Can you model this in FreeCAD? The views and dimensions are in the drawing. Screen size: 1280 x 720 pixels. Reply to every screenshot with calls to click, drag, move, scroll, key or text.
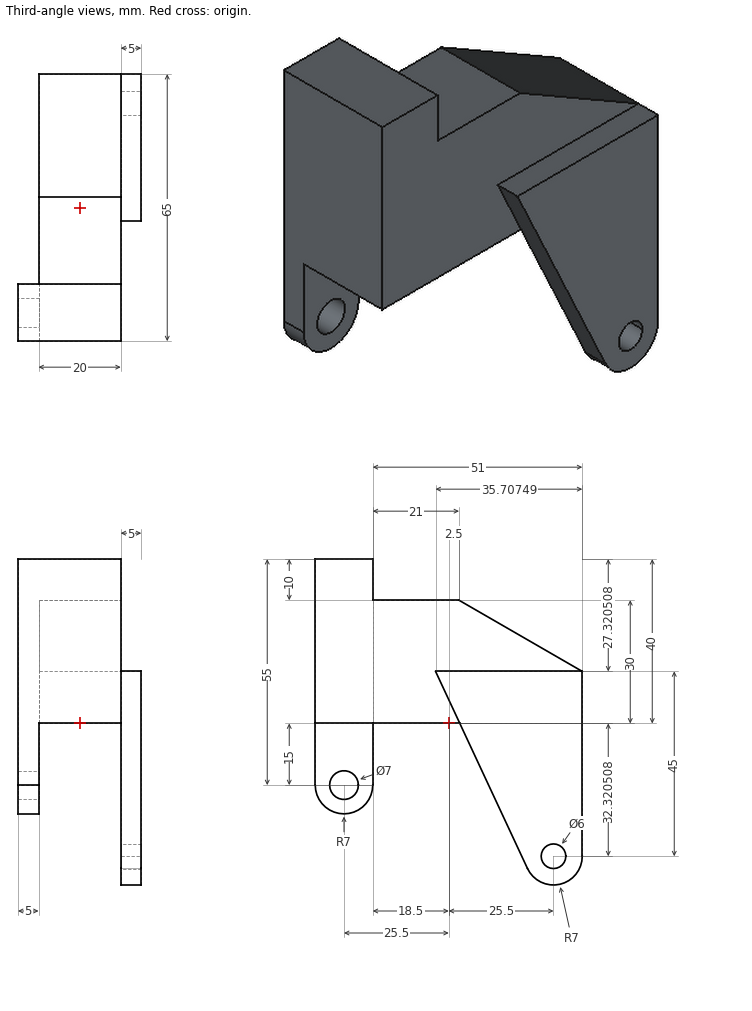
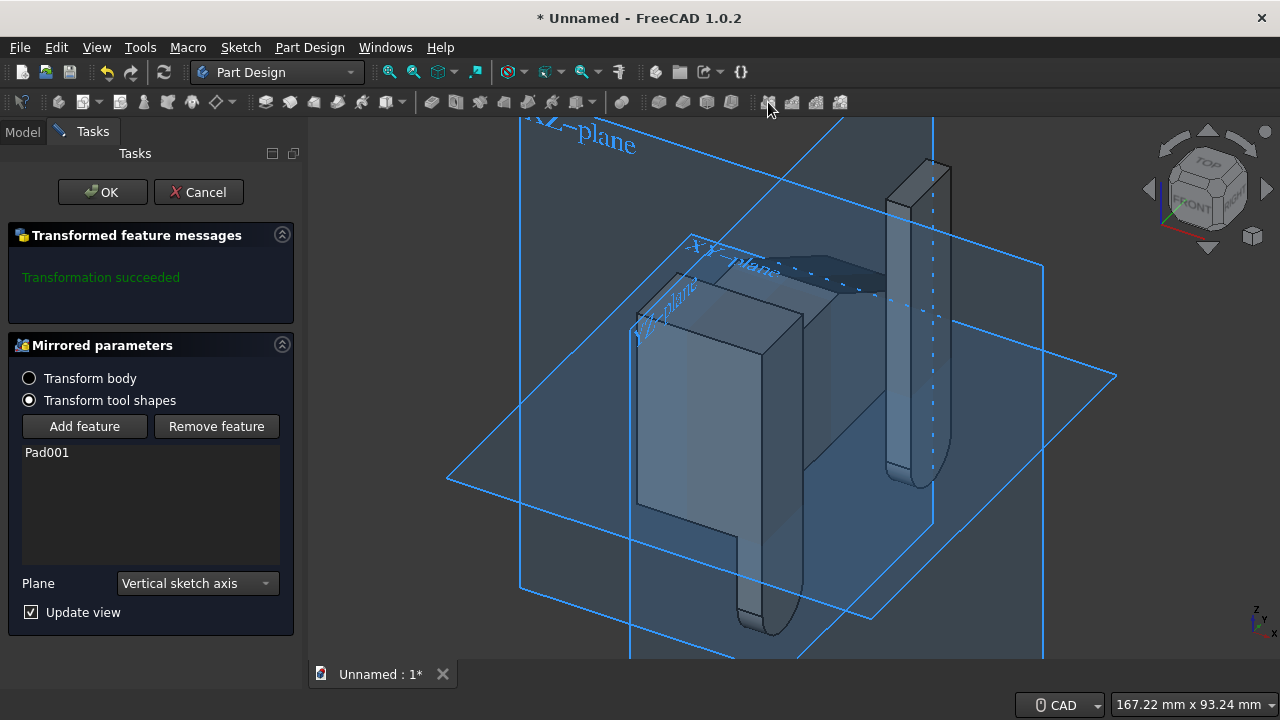
click(198, 584)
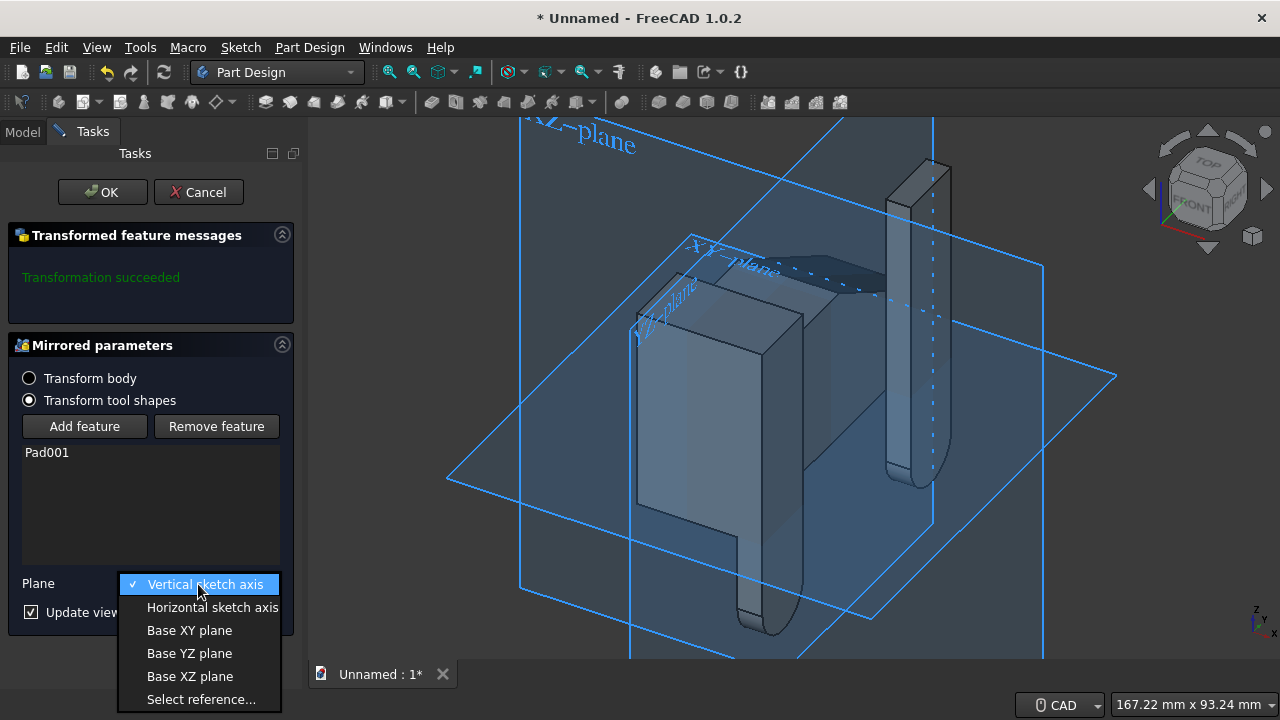
click(198, 654)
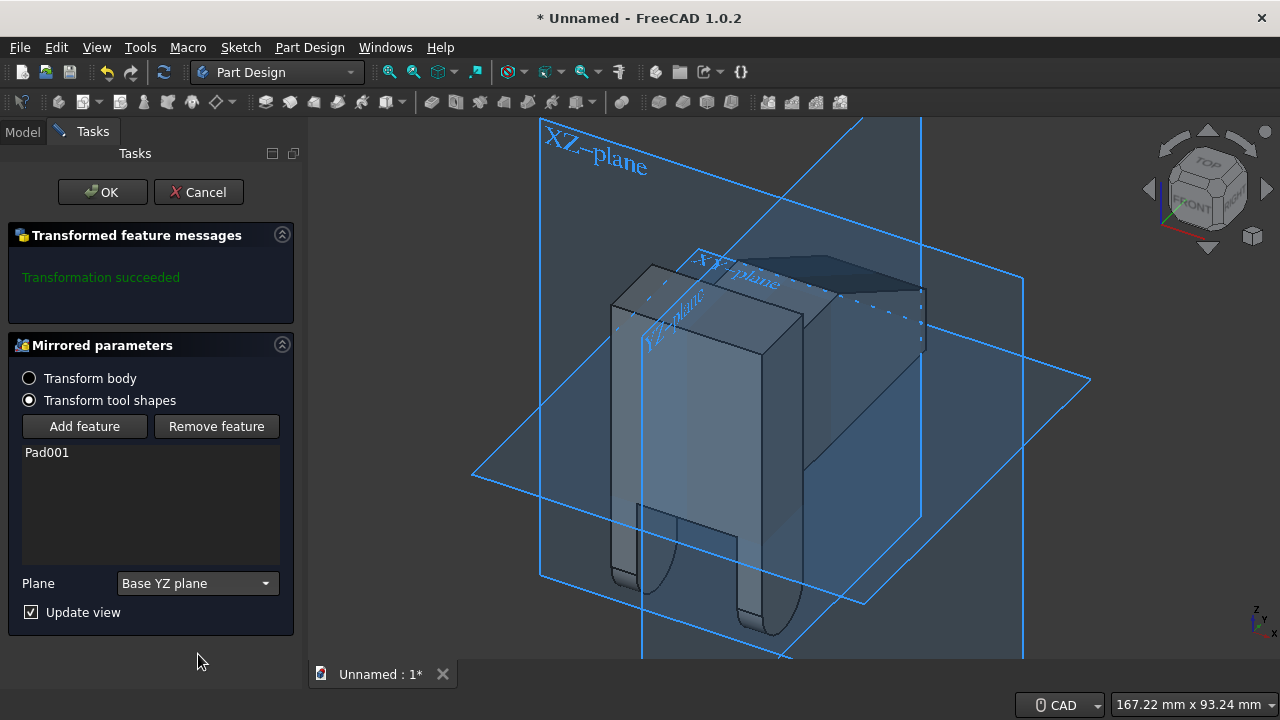
click(103, 192)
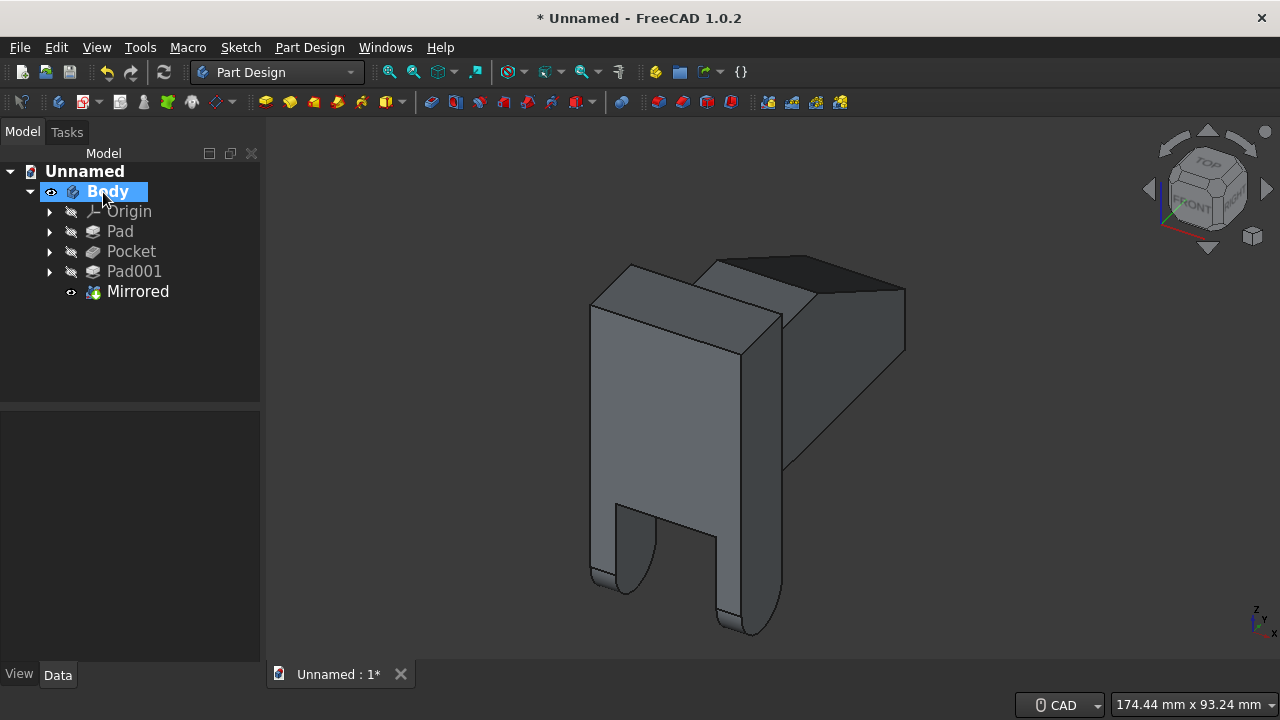
click(390, 72)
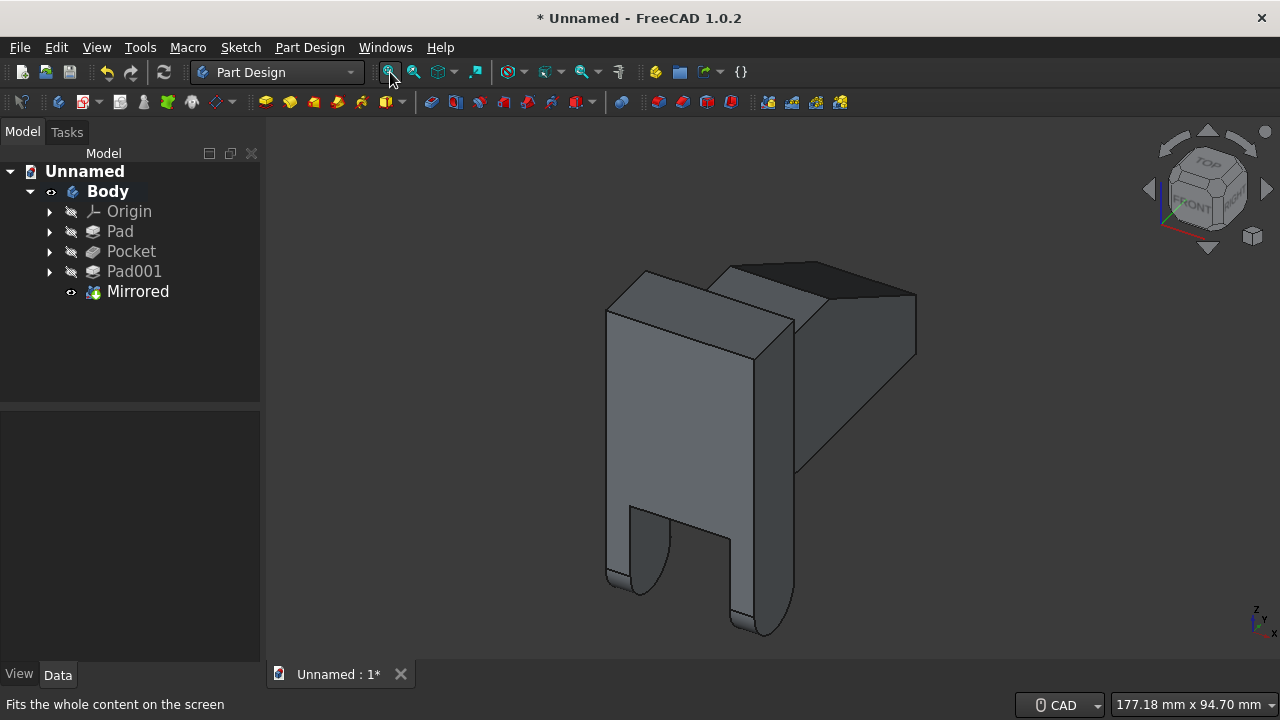
click(774, 401)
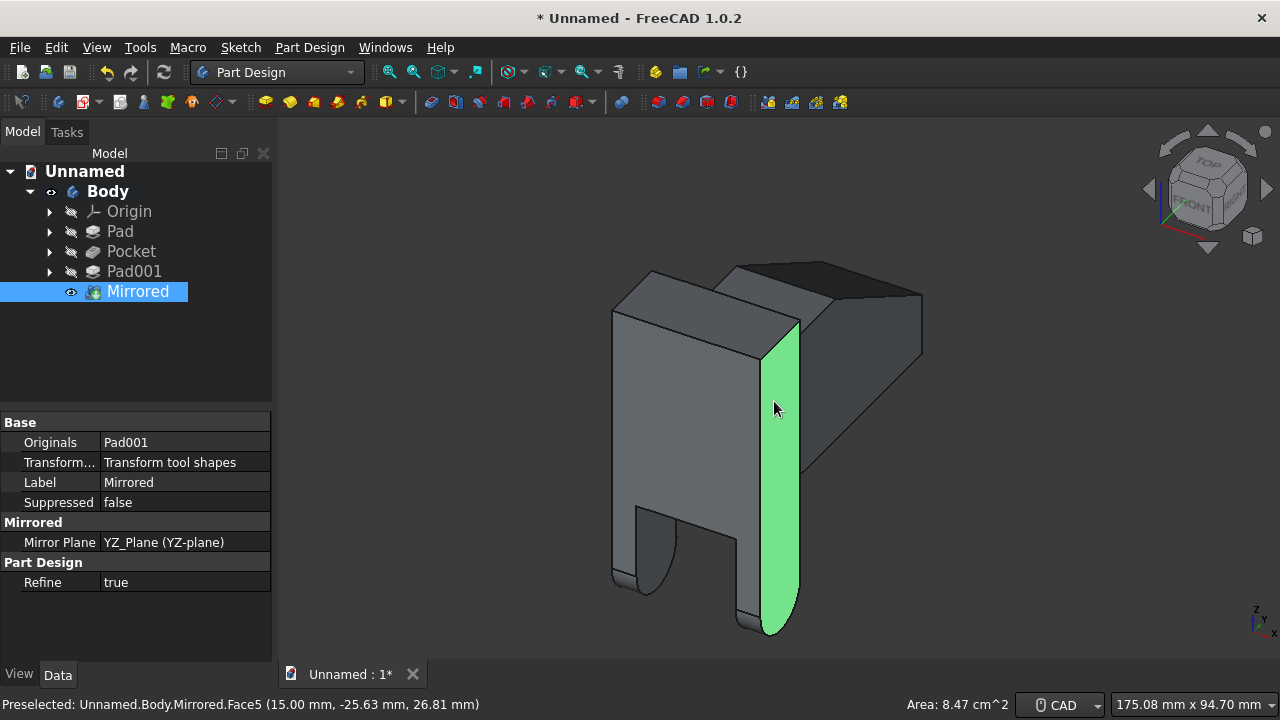
click(84, 102)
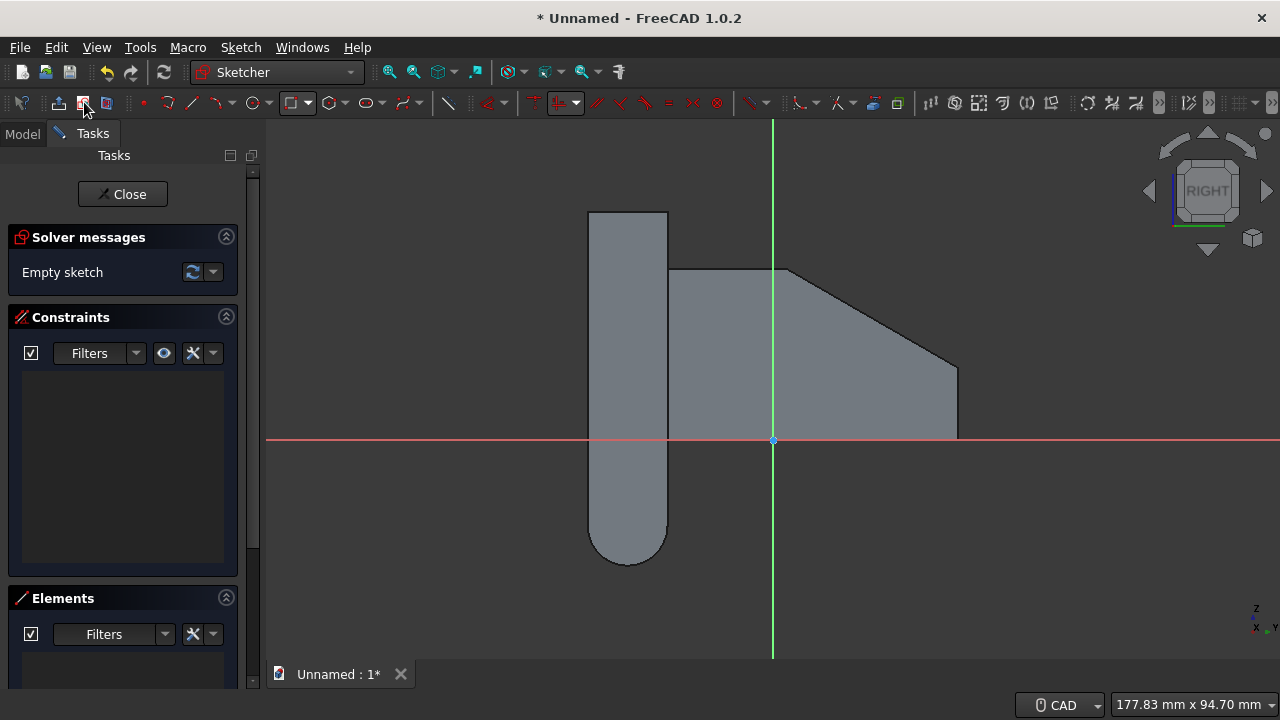
key(g)
key(m)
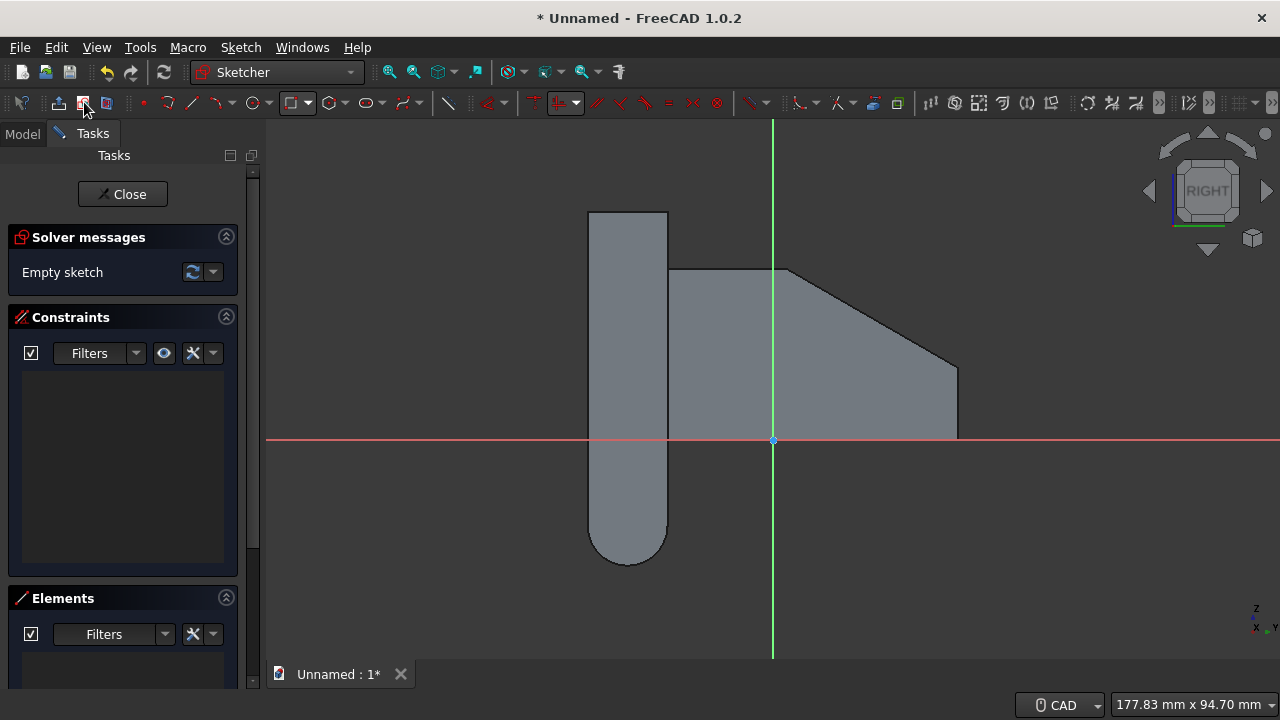
click(668, 526)
click(668, 212)
click(588, 212)
click(588, 526)
right_click(588, 526)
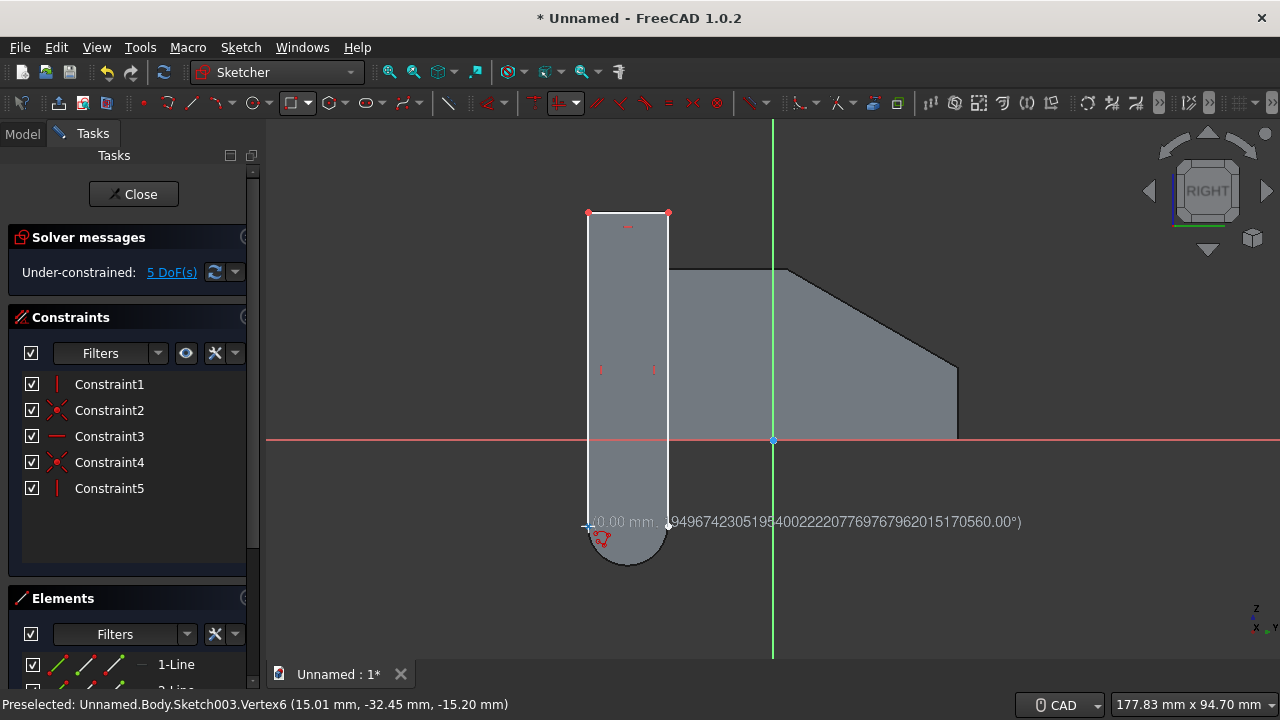
click(216, 104)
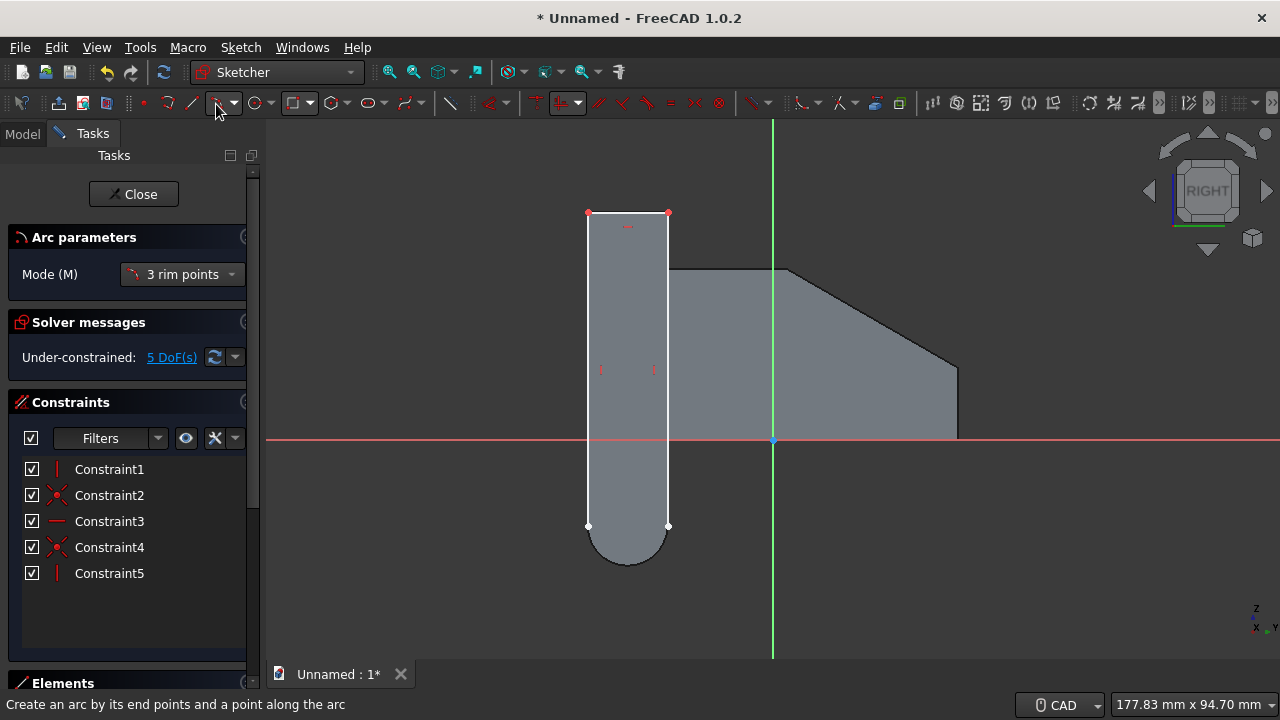
click(588, 527)
click(668, 527)
click(628, 566)
key(Escape)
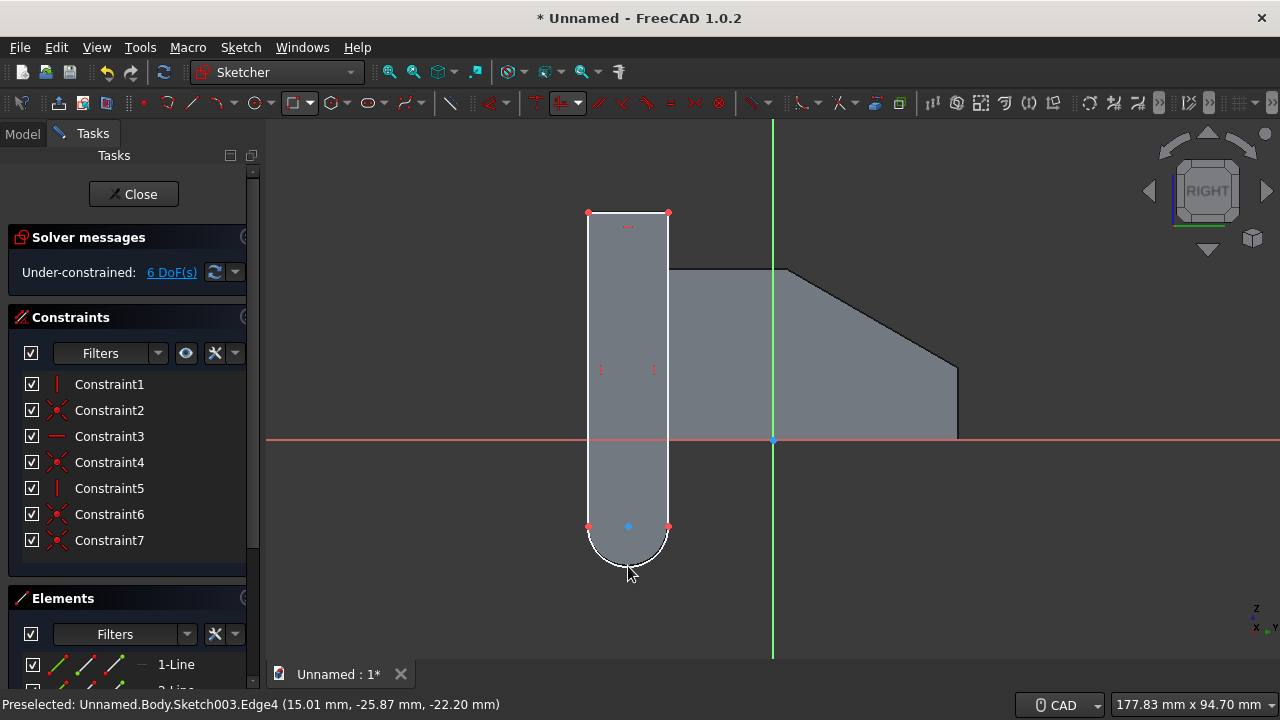
click(668, 307)